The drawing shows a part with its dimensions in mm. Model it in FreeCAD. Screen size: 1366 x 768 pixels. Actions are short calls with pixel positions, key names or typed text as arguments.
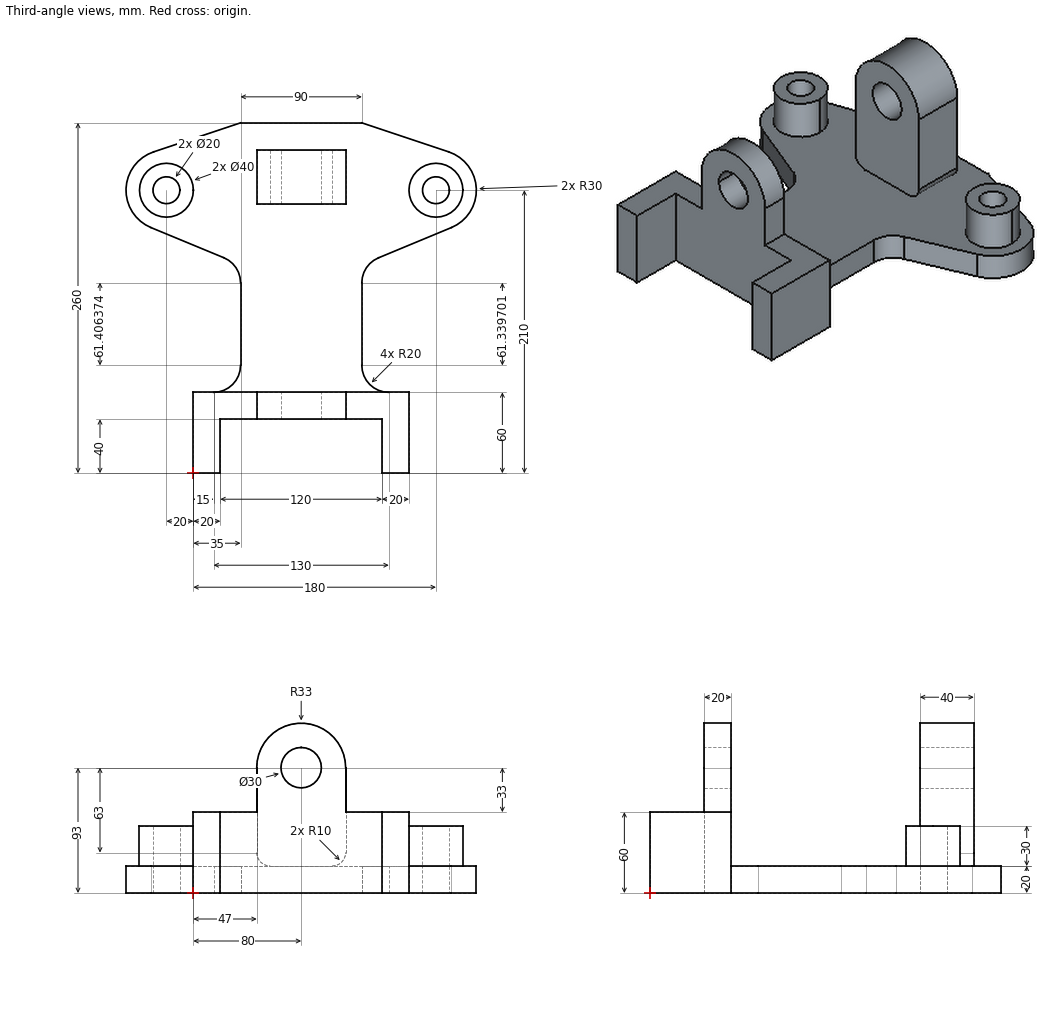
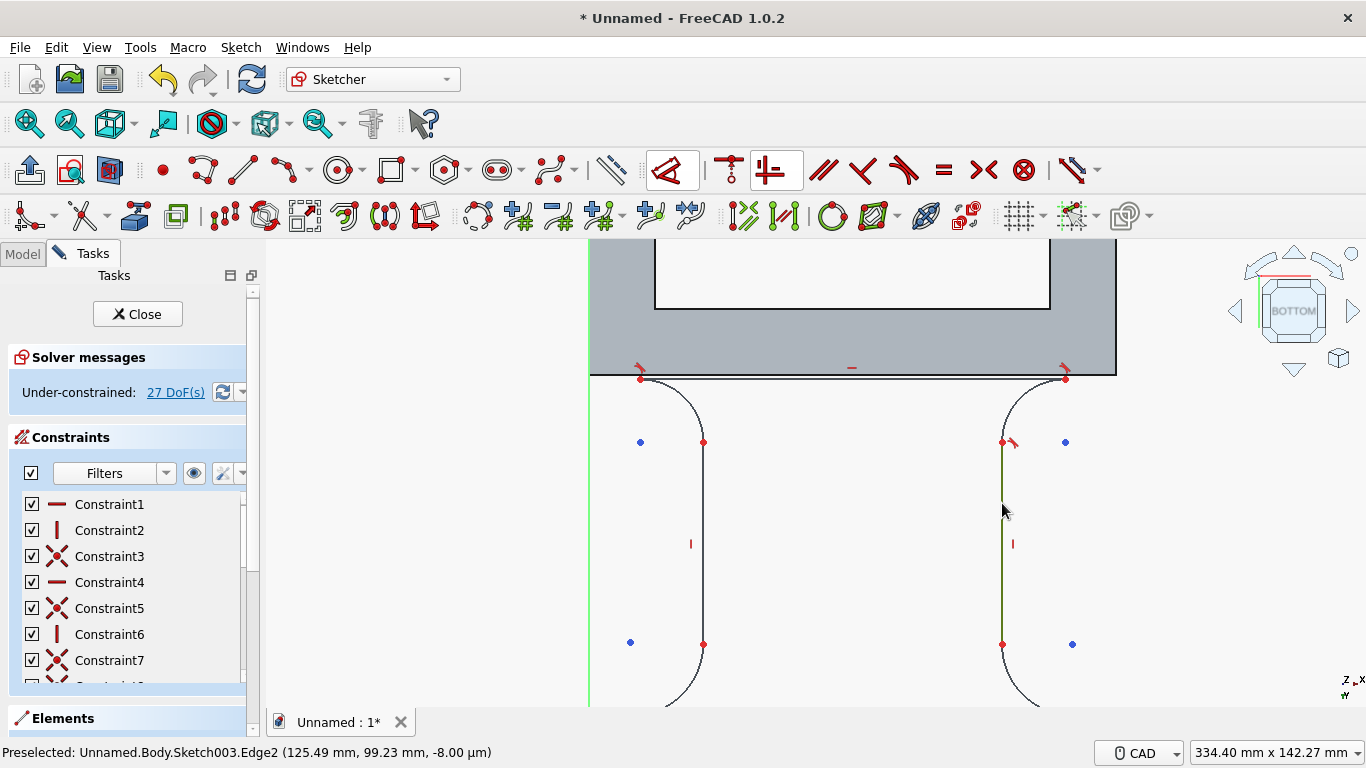
click(1006, 668)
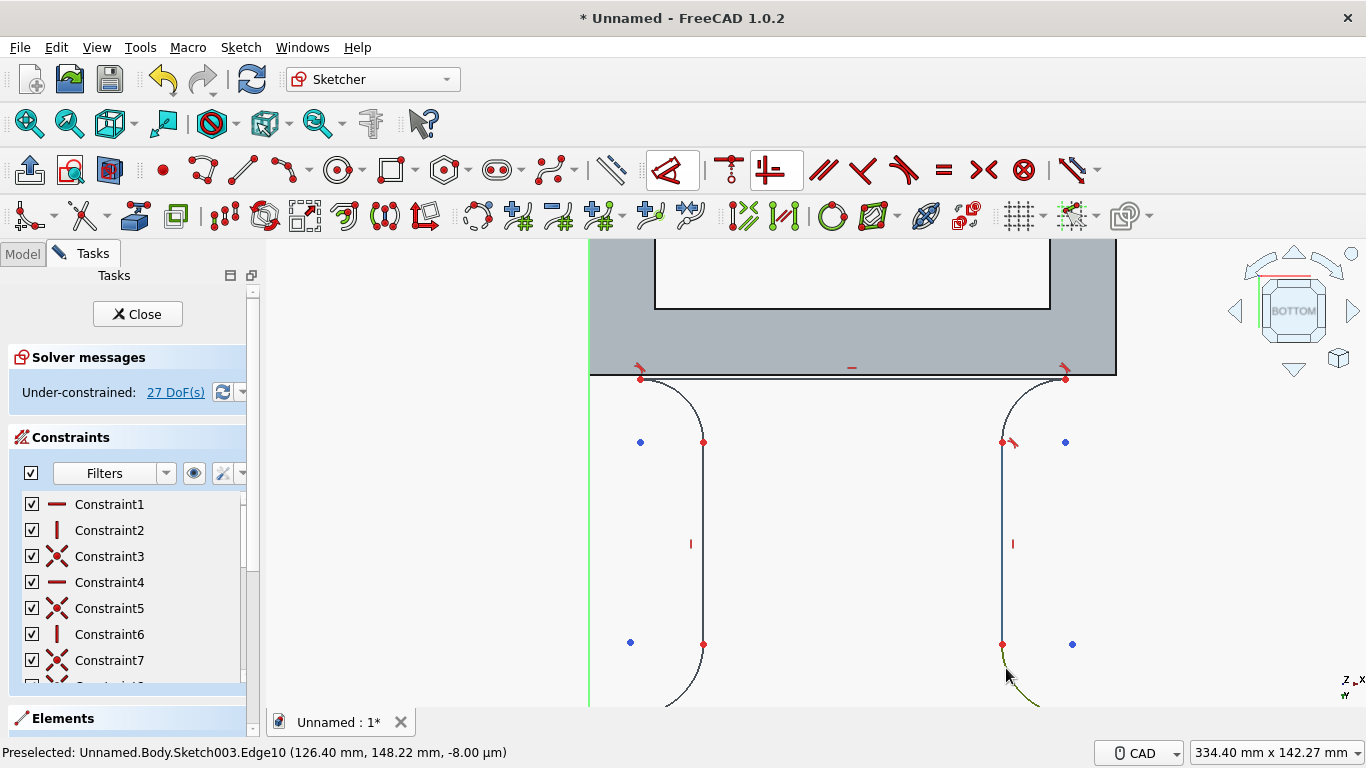
click(904, 170)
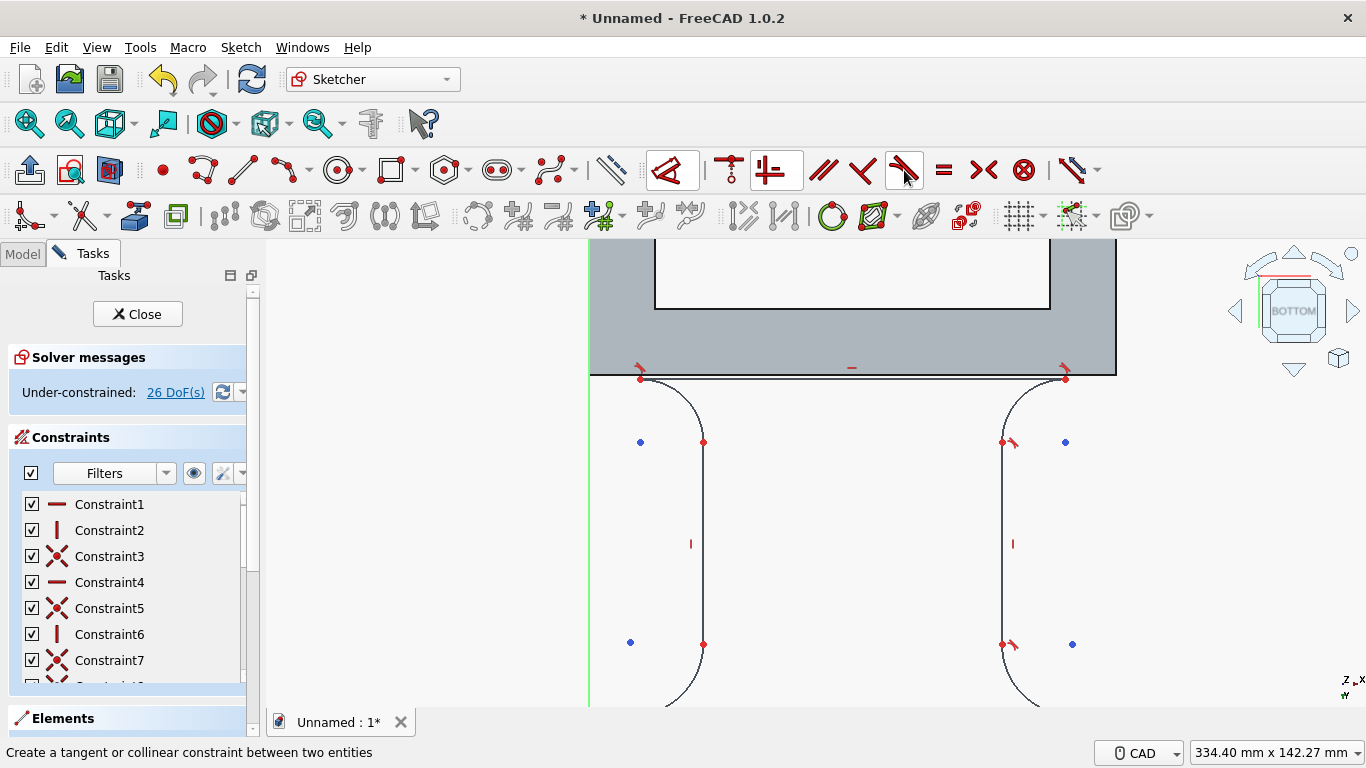
scroll(686, 396, down, 5)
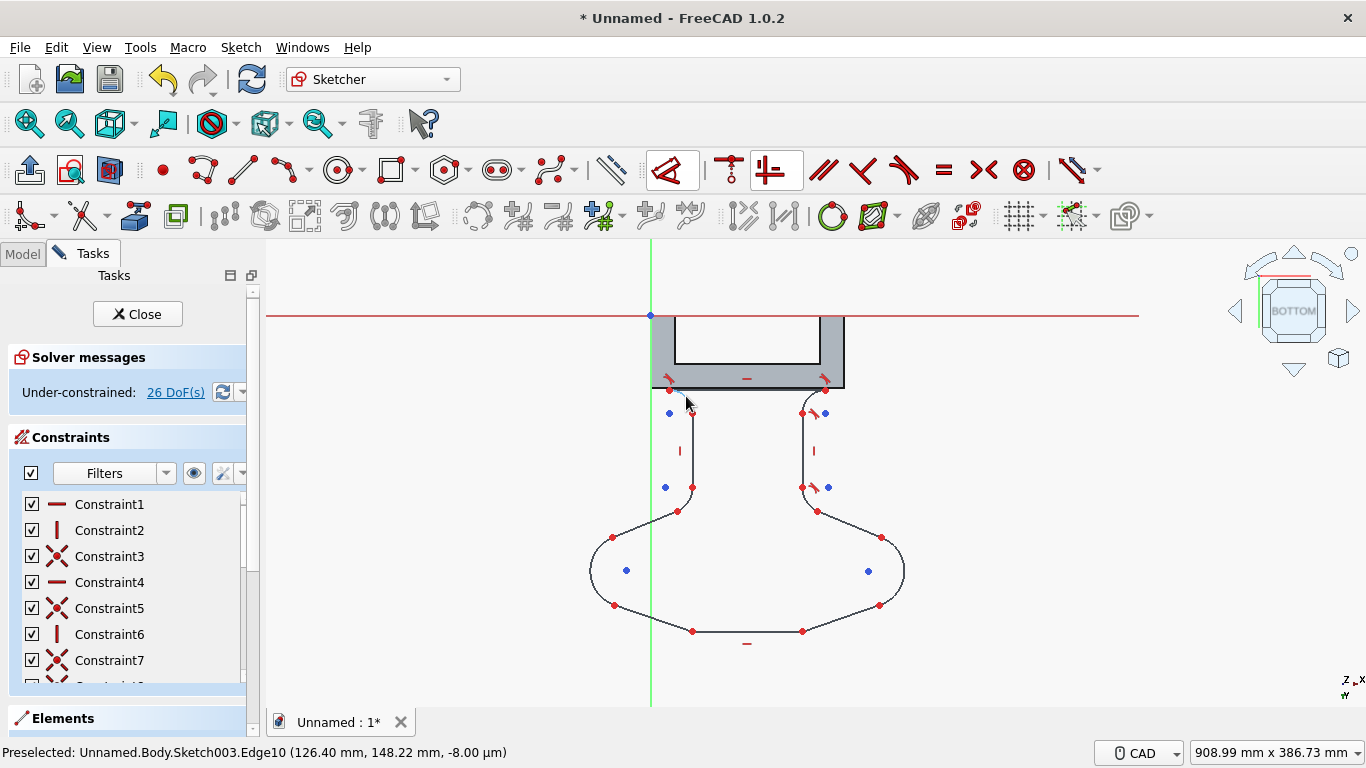
click(837, 519)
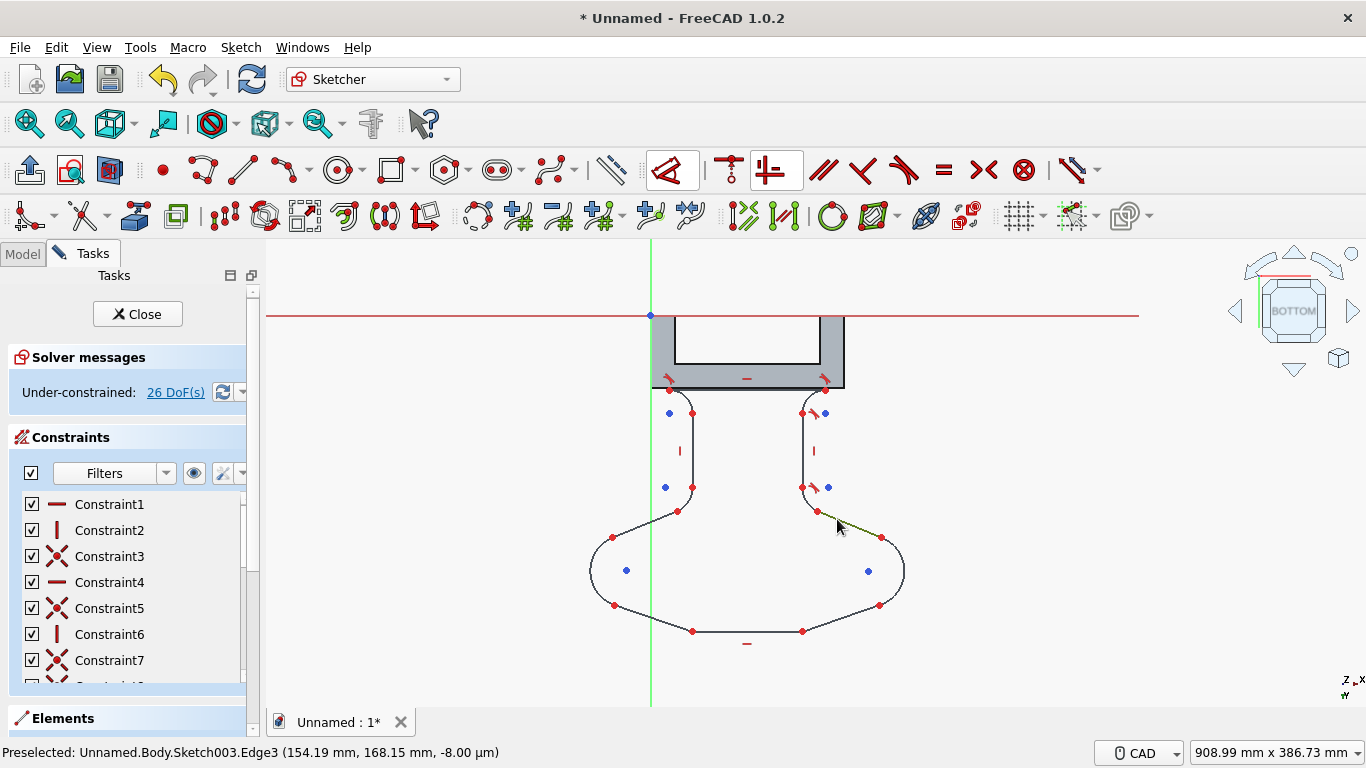
click(807, 502)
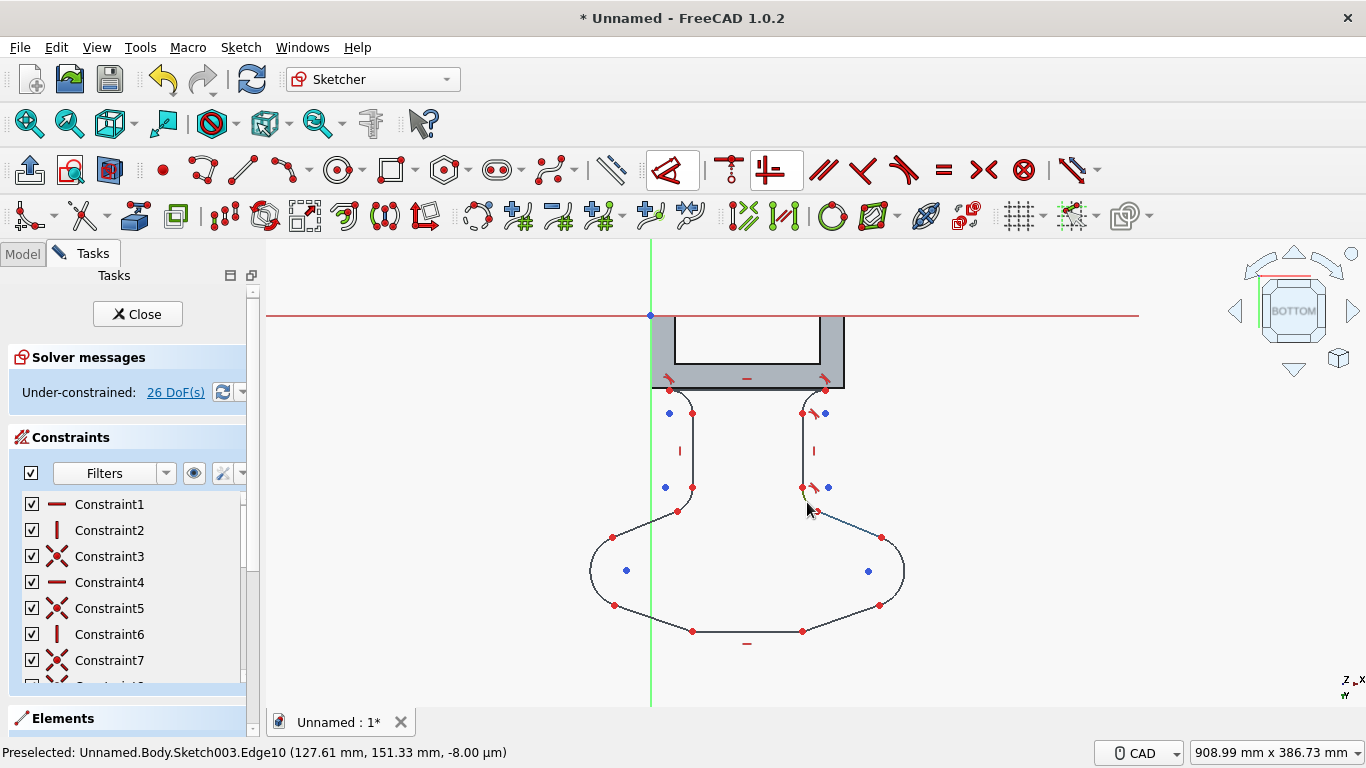
key(t)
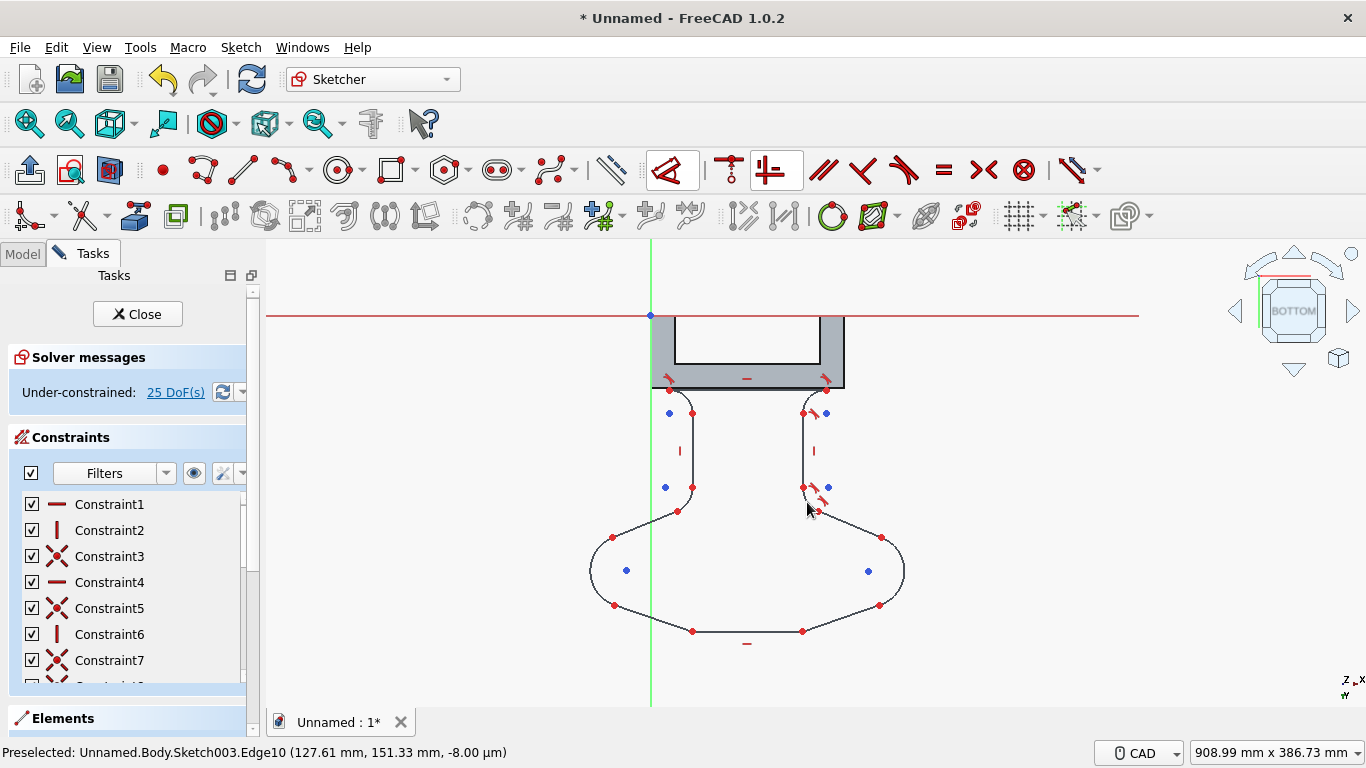
click(837, 519)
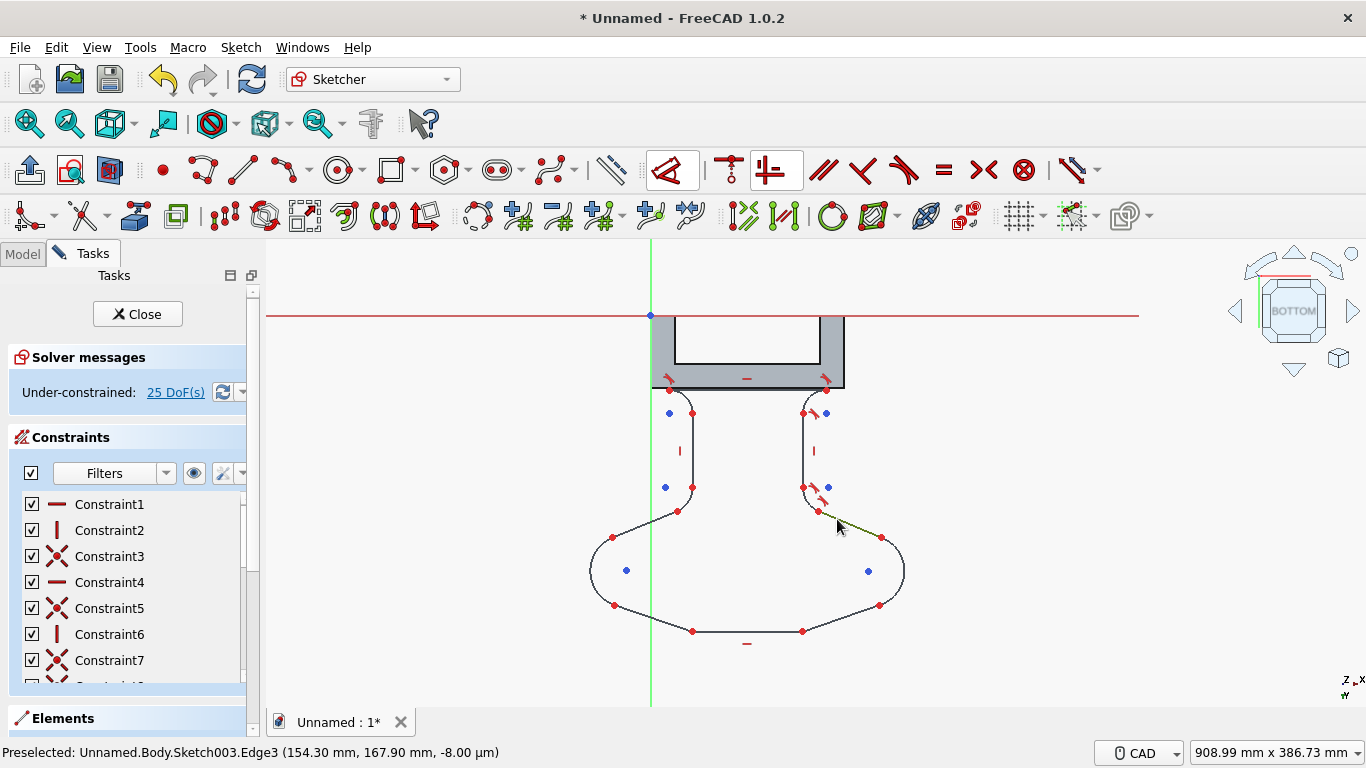
click(900, 589)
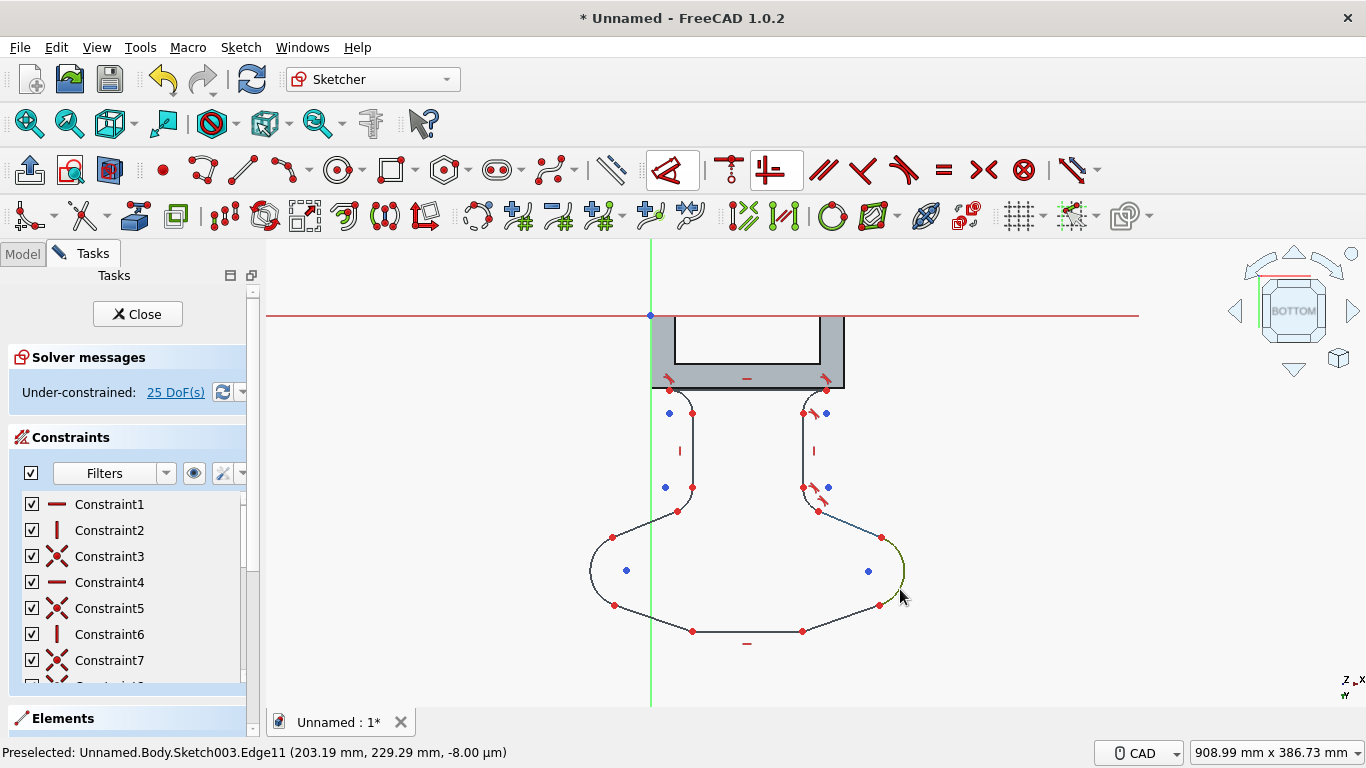
click(904, 170)